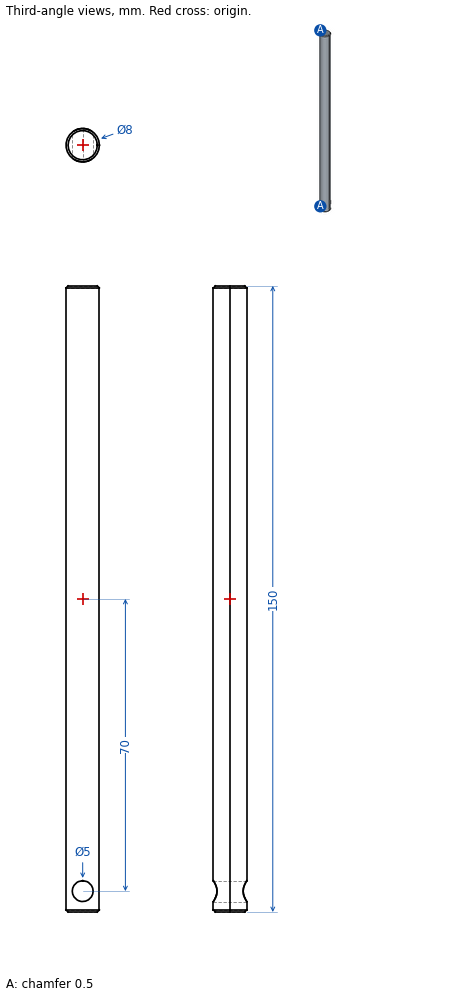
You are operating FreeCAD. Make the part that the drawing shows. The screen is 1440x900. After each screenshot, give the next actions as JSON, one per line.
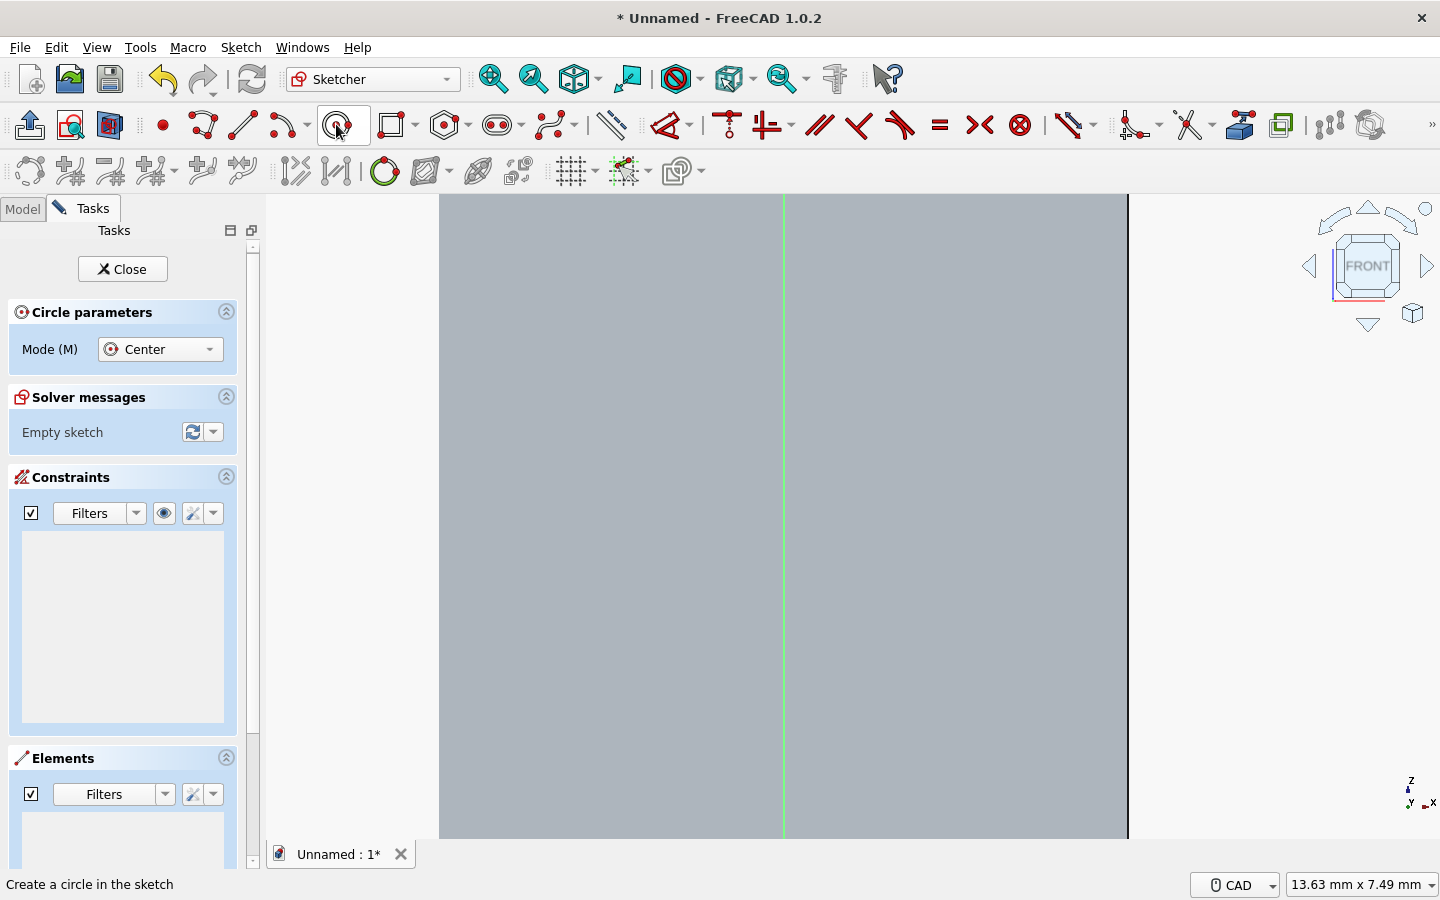
{"action": "left_click", "coordinate": [784, 515]}
{"action": "left_click", "coordinate": [936, 363]}
{"action": "key", "text": "Escape"}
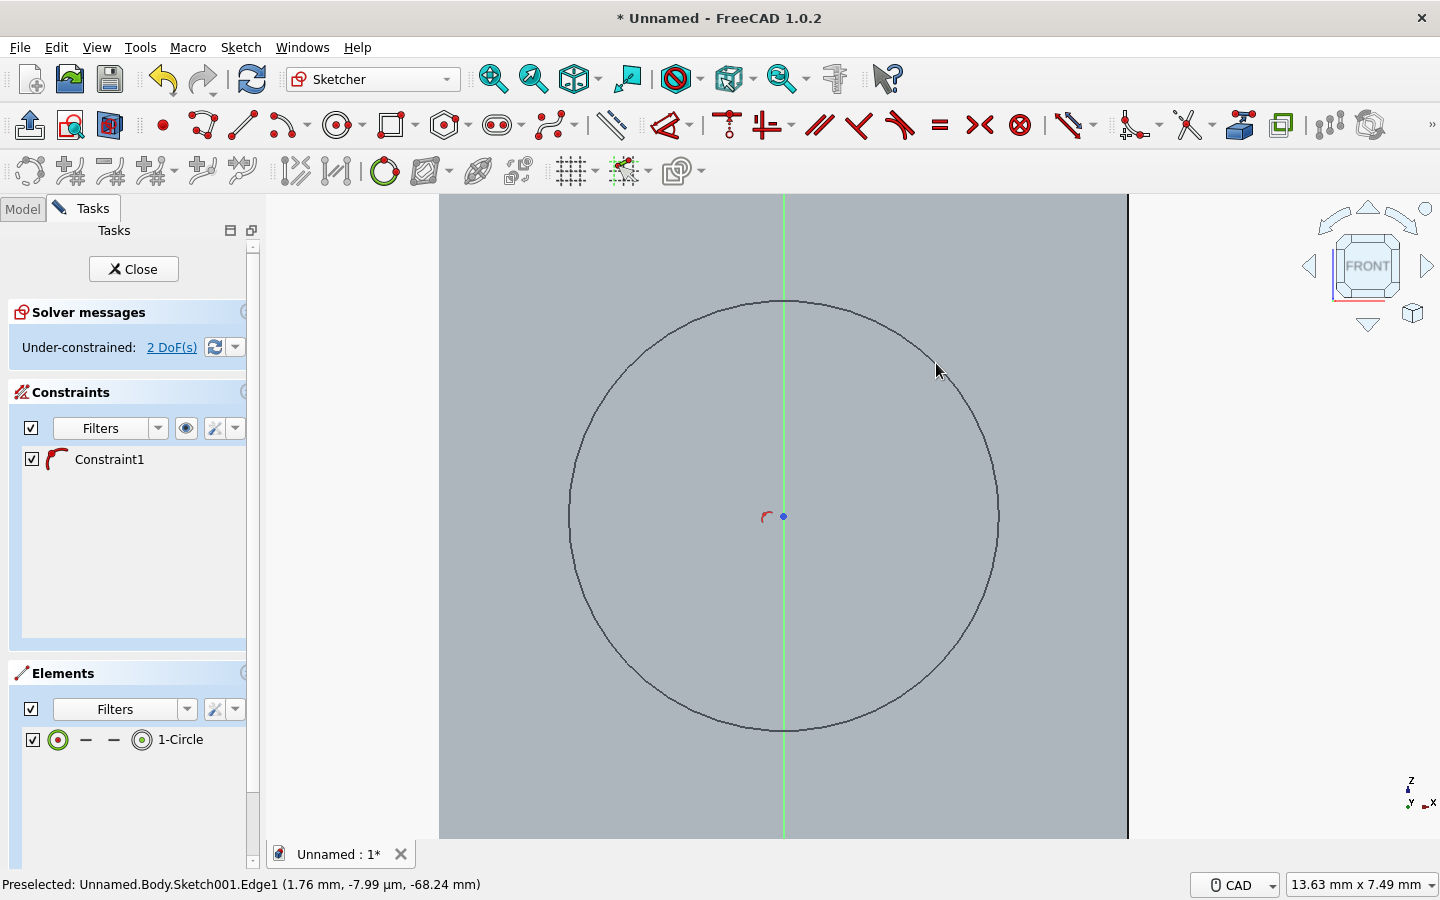
{"action": "left_click", "coordinate": [666, 126]}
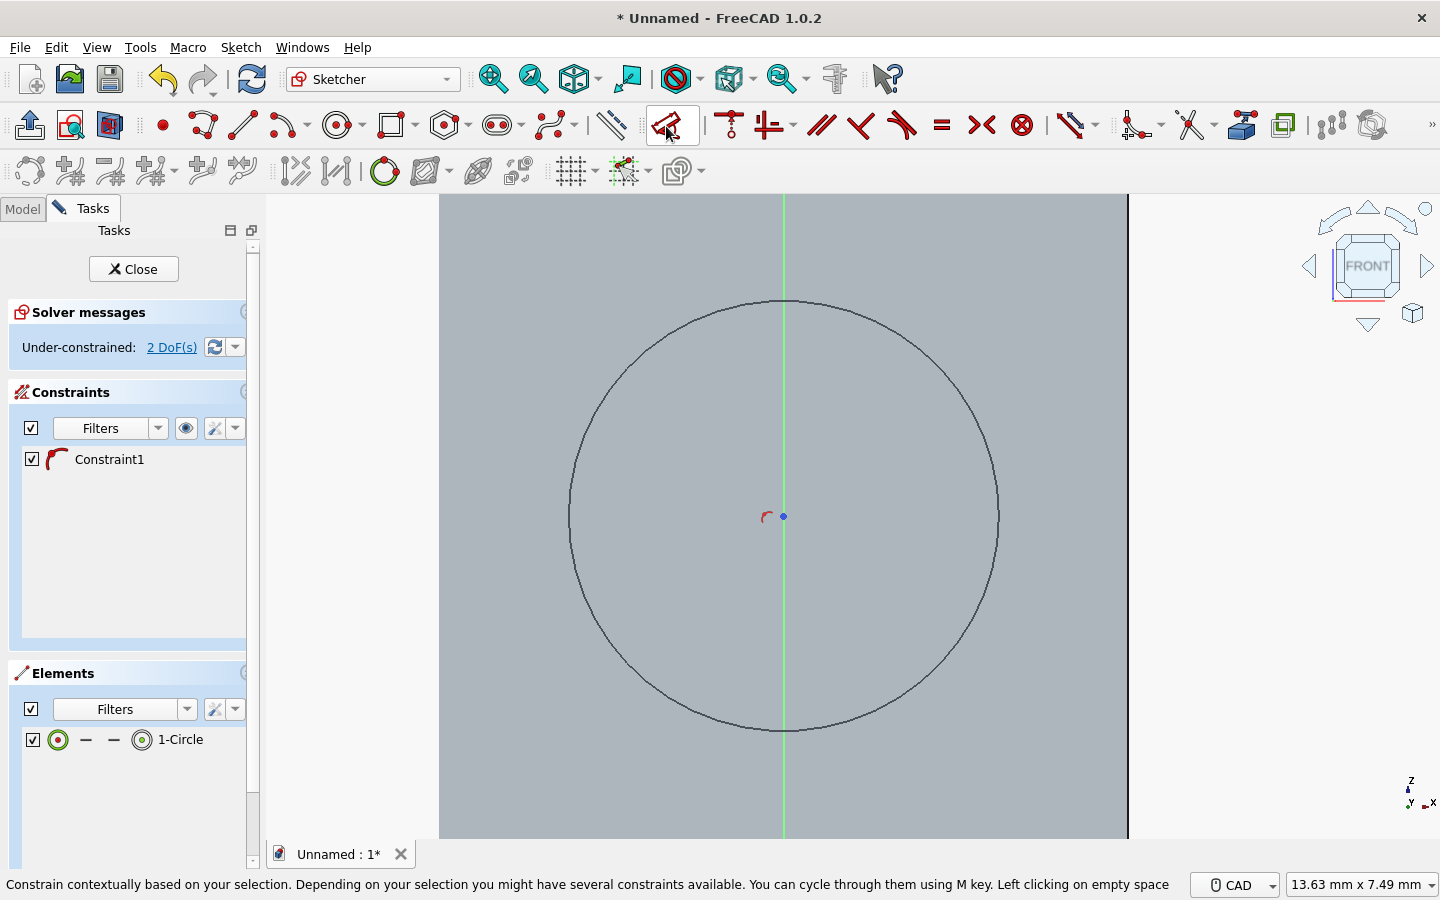
{"action": "left_click", "coordinate": [935, 363]}
{"action": "left_click", "coordinate": [957, 340]}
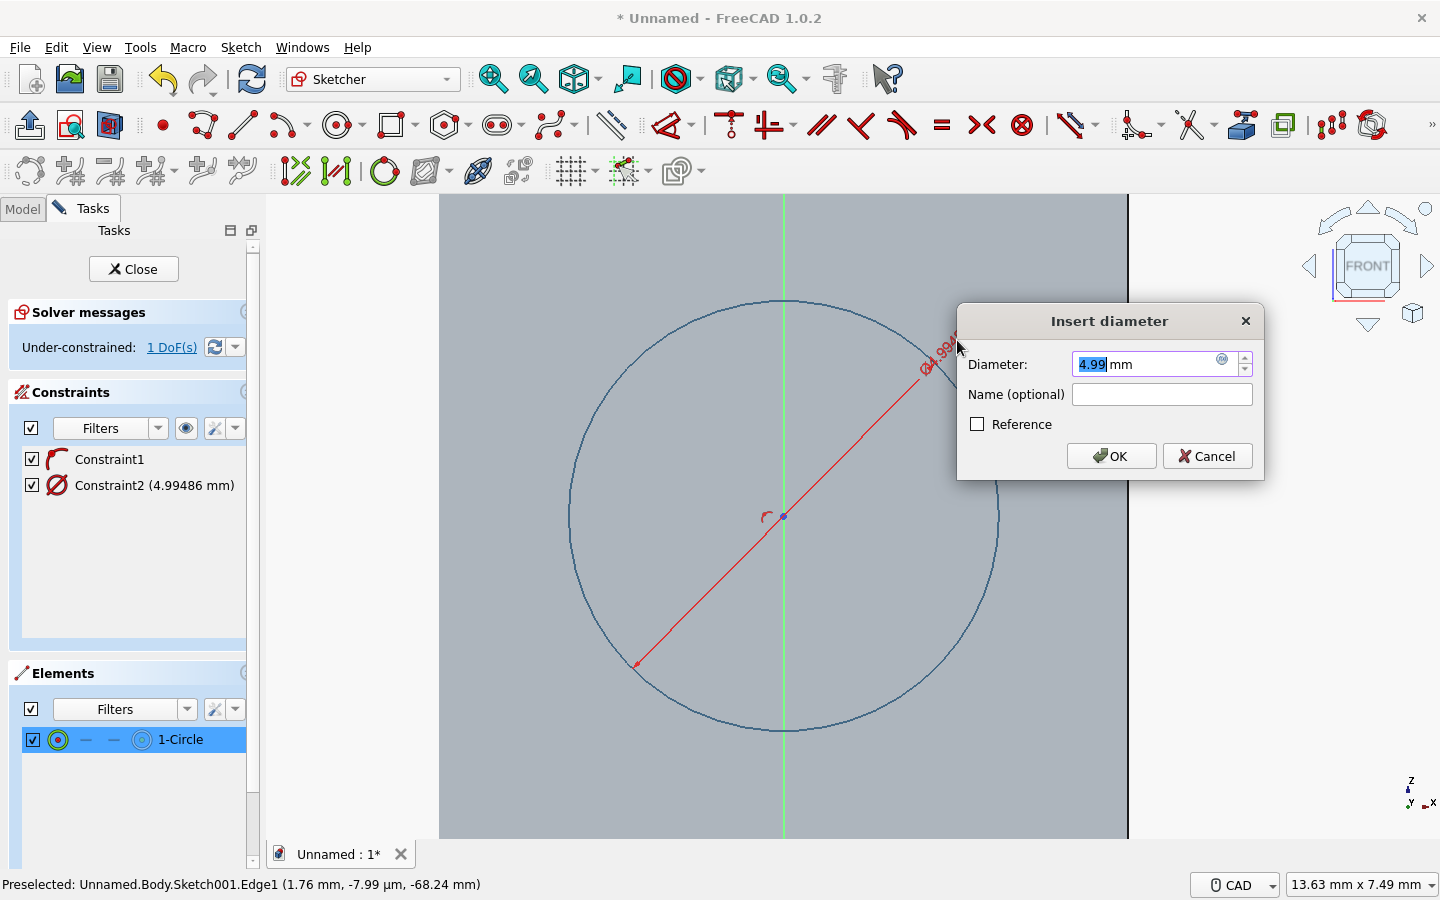
{"action": "type", "text": "5"}
{"action": "key", "text": "Return"}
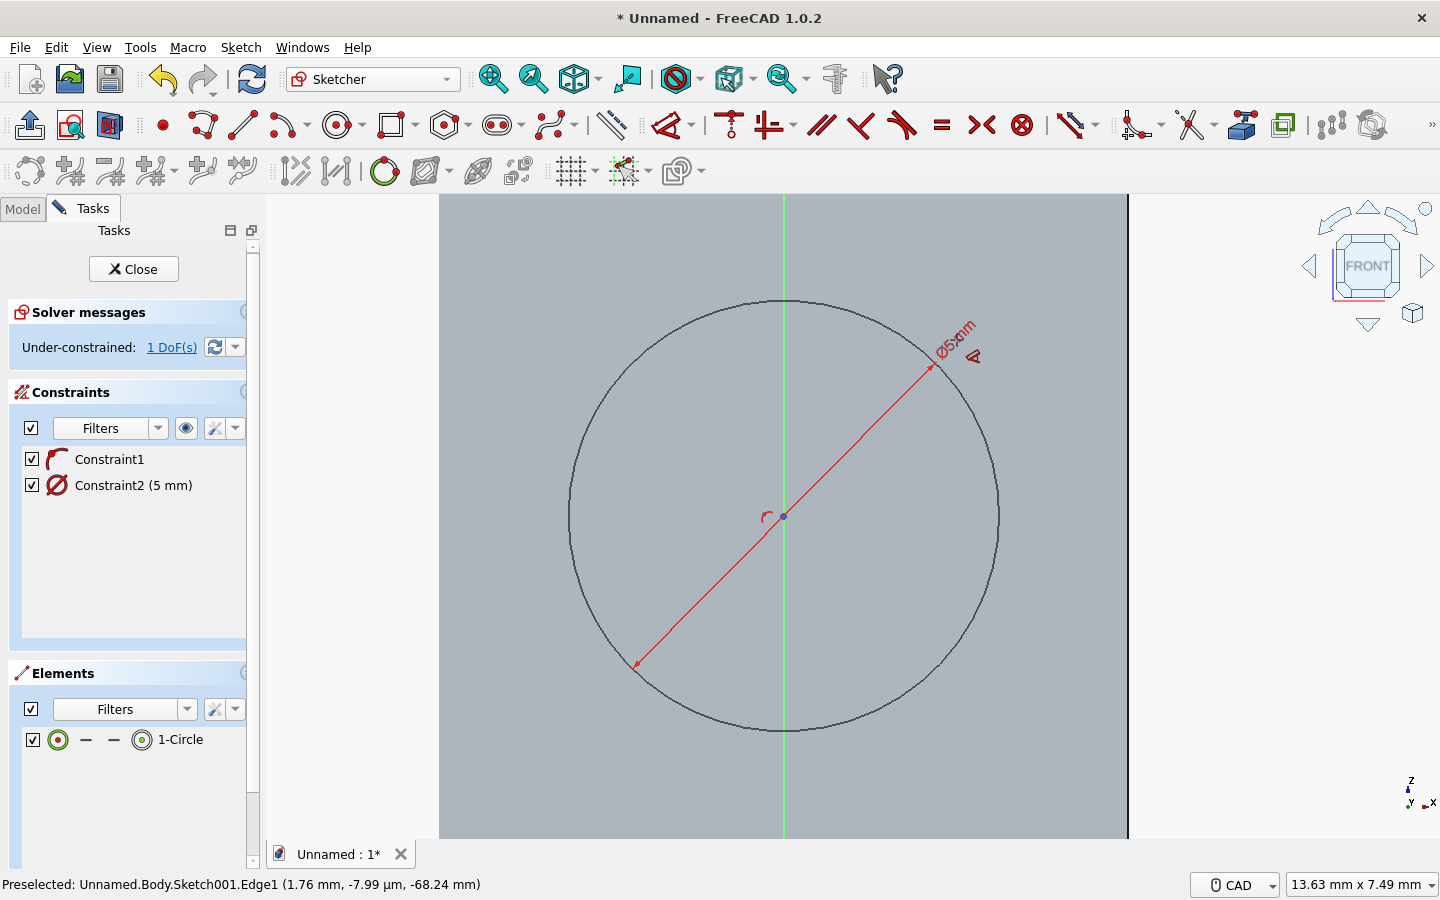
{"action": "left_click", "coordinate": [784, 516]}
{"action": "left_click", "coordinate": [818, 369]}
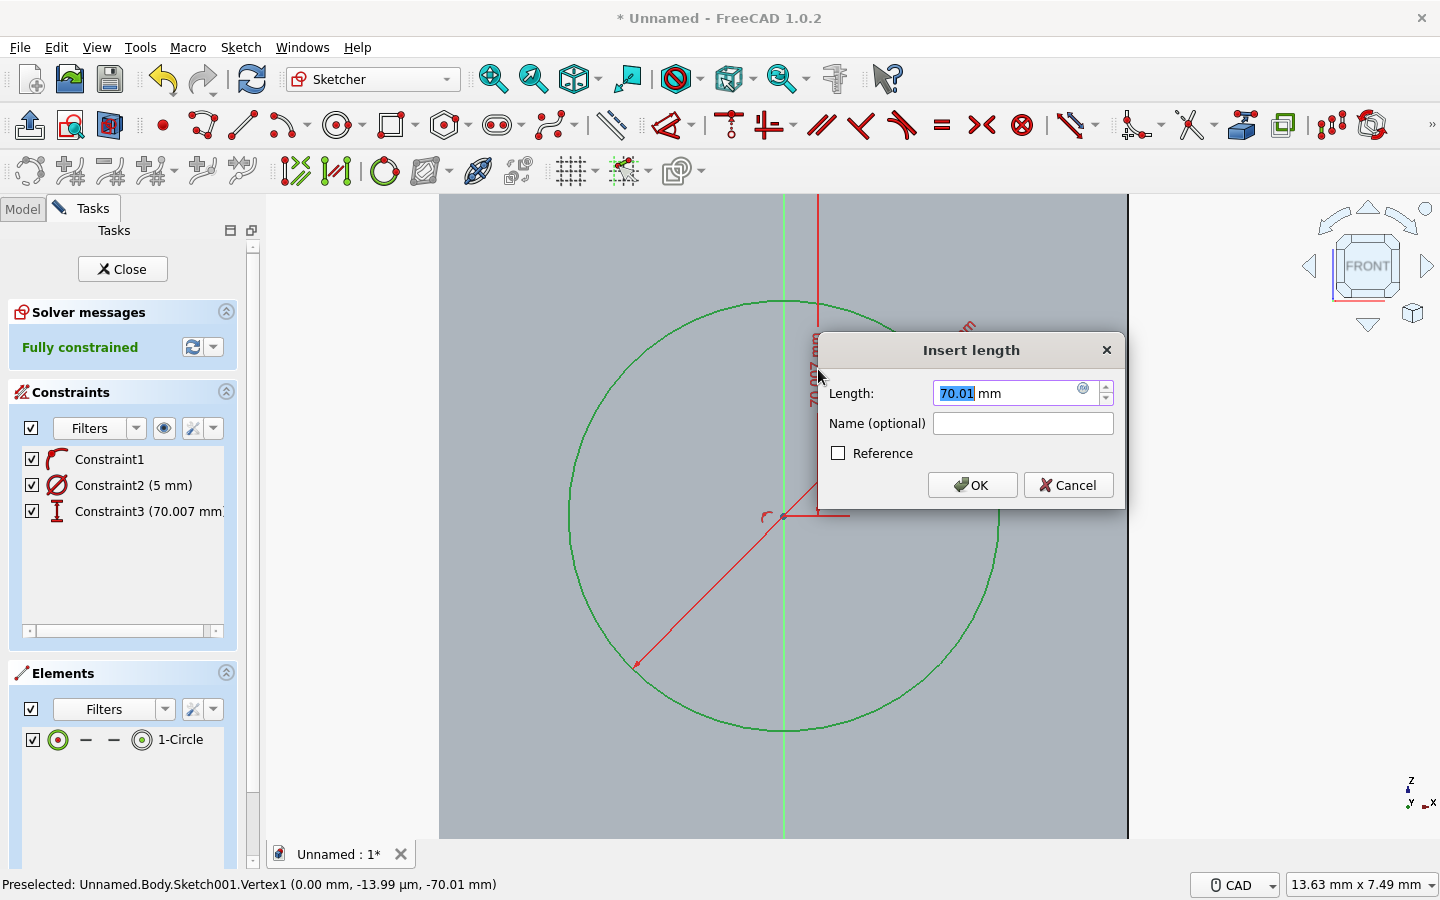
{"action": "type", "text": "70"}
{"action": "key", "text": "Return"}
{"action": "key", "text": "Escape"}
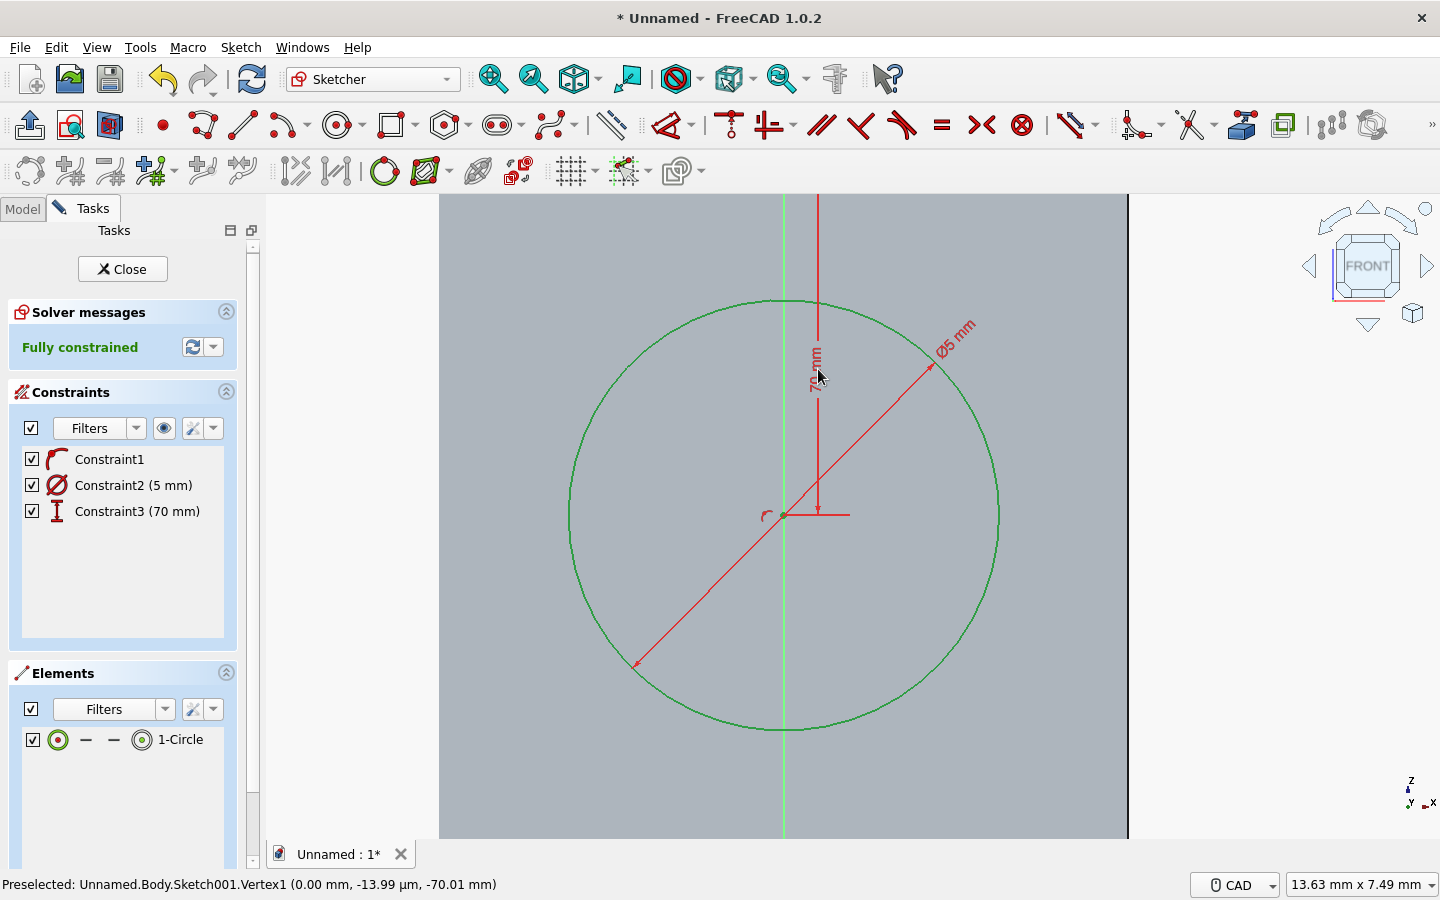
{"action": "left_click", "coordinate": [123, 269]}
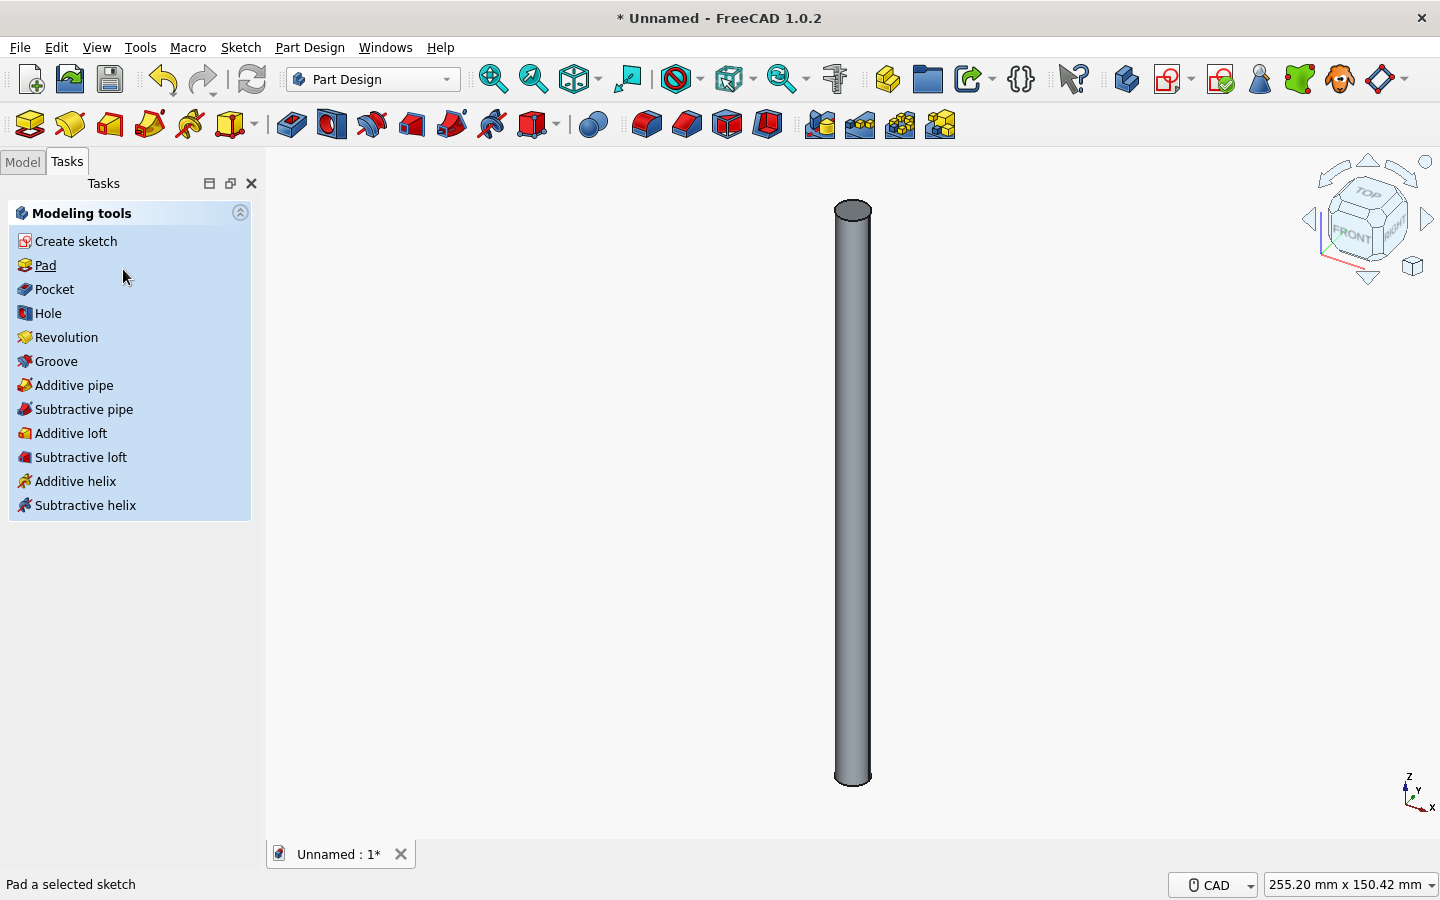
{"action": "left_click", "coordinate": [292, 124]}